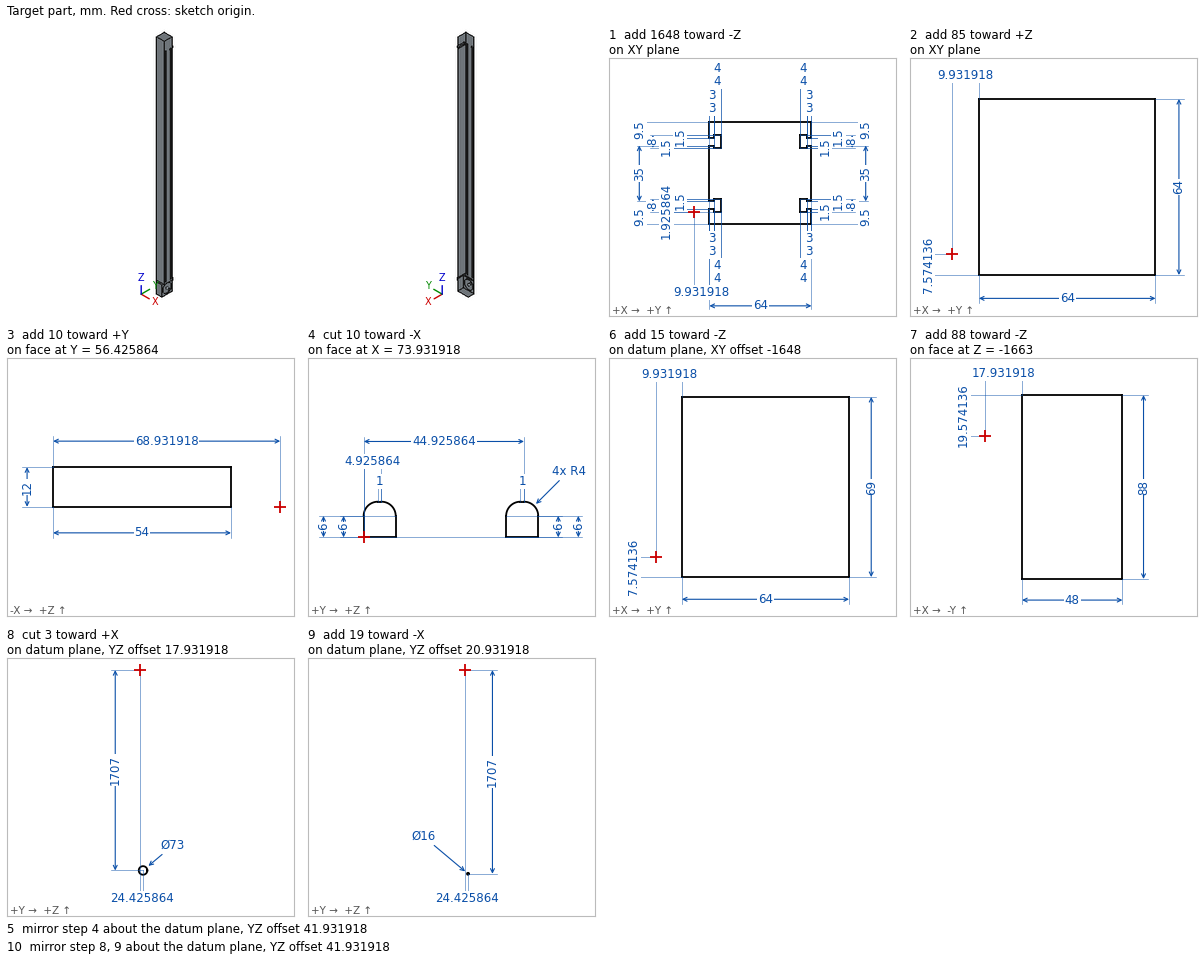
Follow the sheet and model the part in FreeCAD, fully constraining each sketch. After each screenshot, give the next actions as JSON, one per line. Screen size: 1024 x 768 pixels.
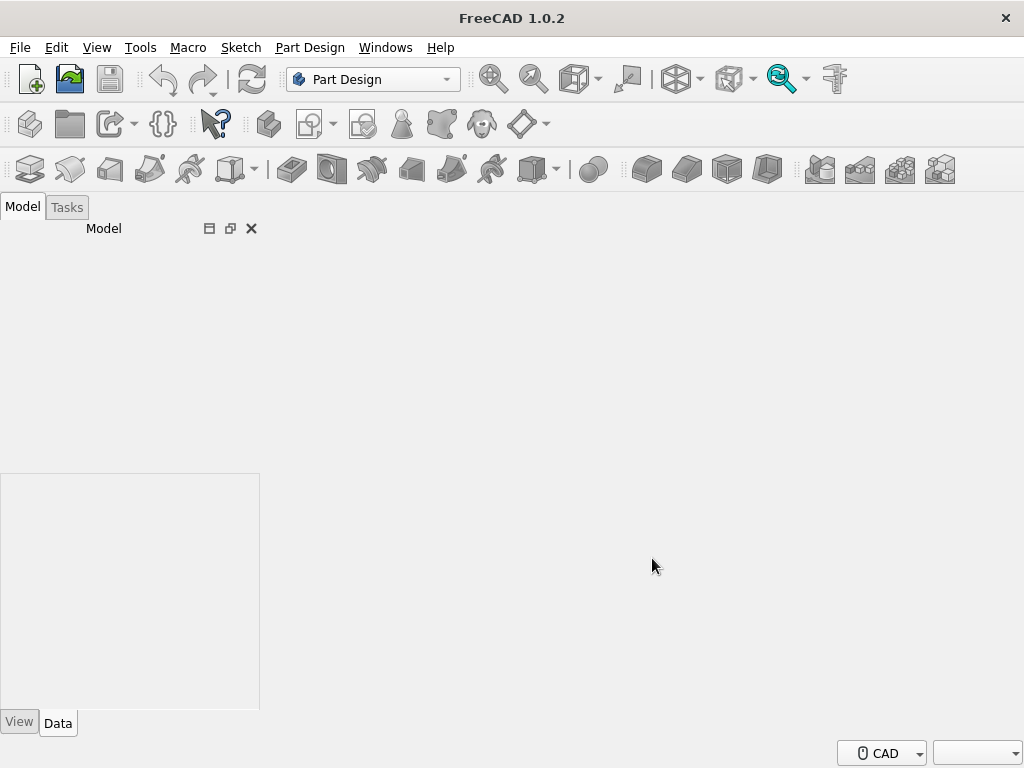
{"action": "left_click", "coordinate": [30, 80]}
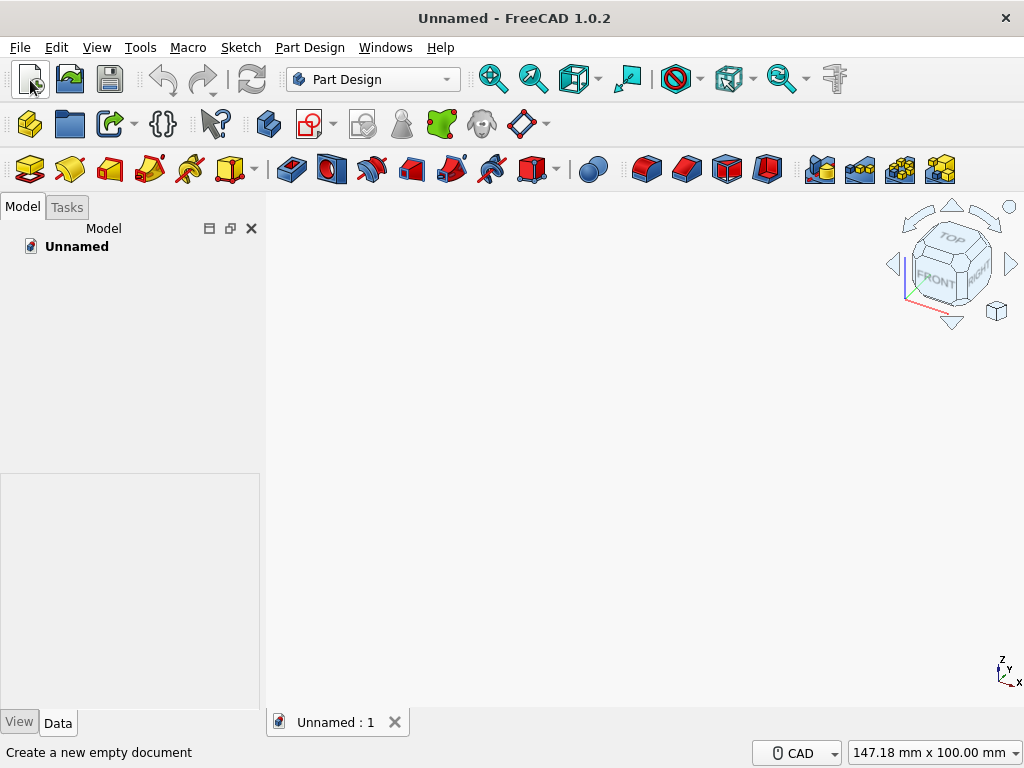
{"action": "left_click", "coordinate": [310, 124]}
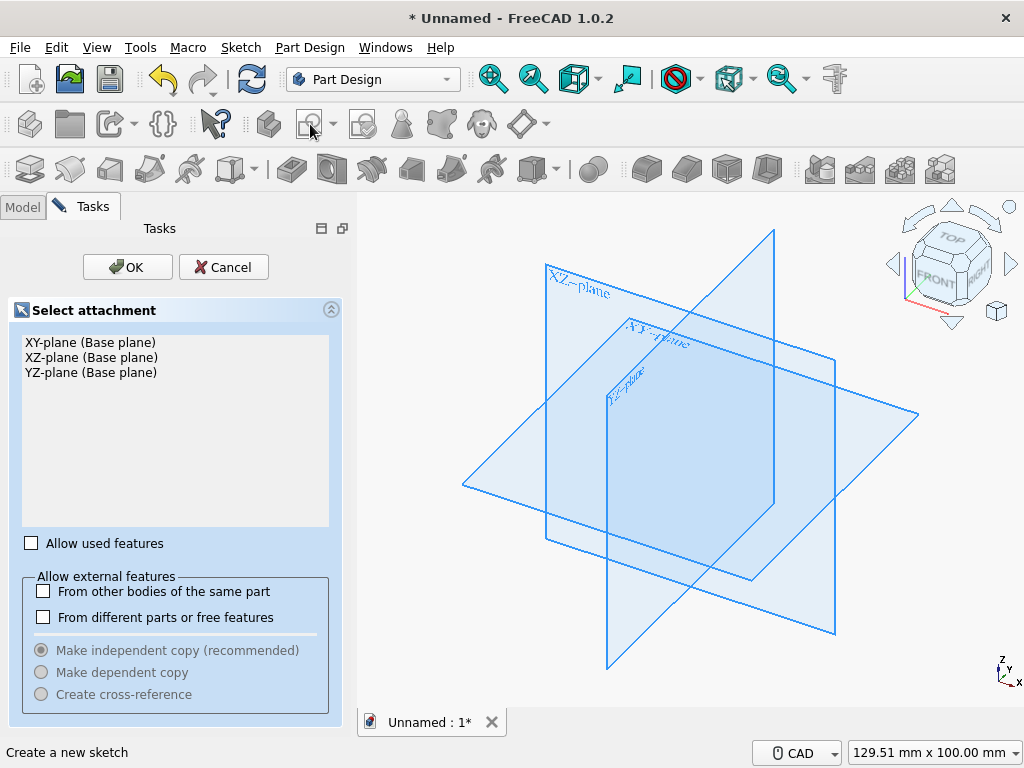
{"action": "left_click", "coordinate": [82, 342]}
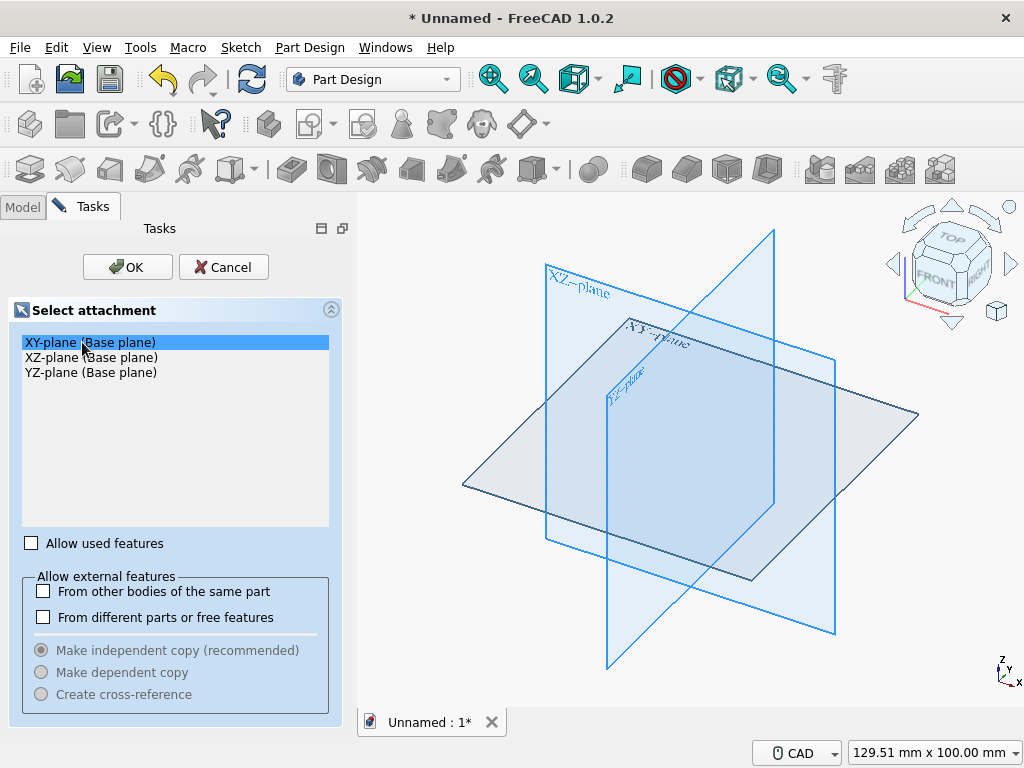
{"action": "left_click", "coordinate": [128, 267]}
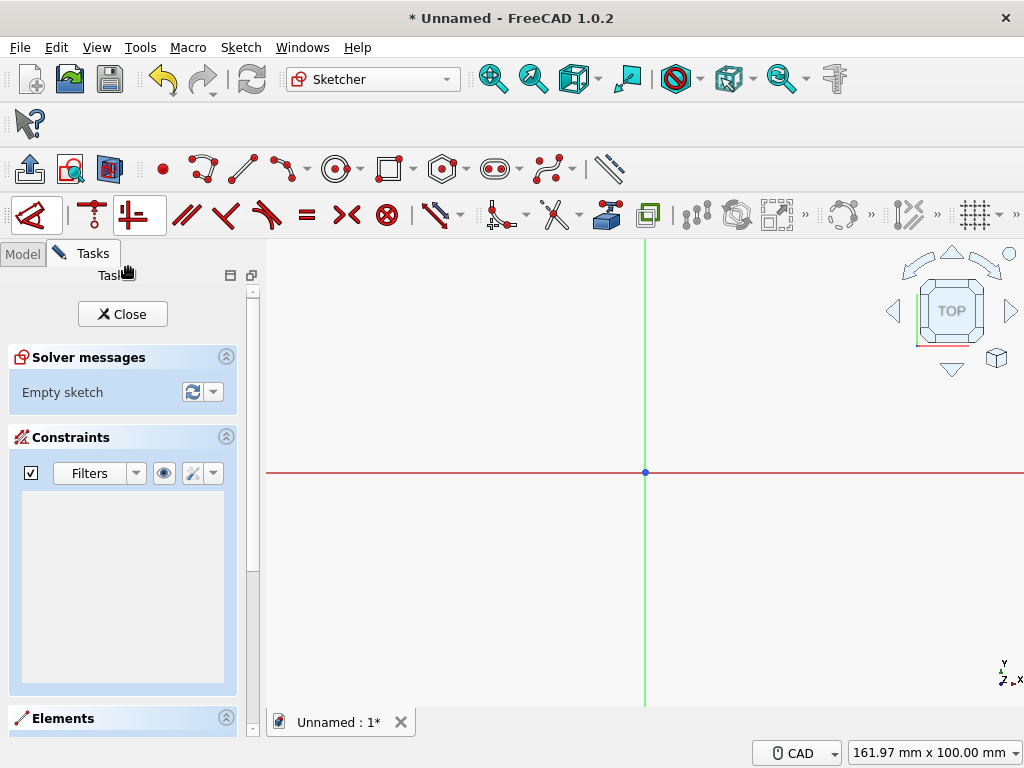
{"action": "scroll", "coordinate": [294, 679], "scroll_direction": "down", "scroll_amount": 2}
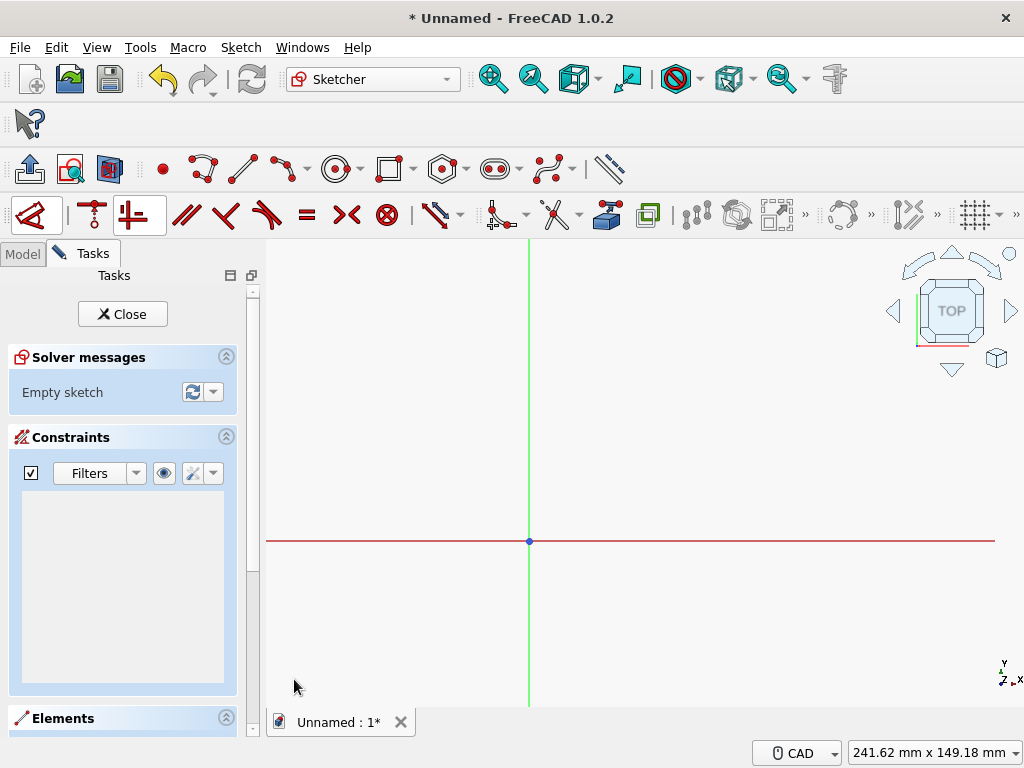
{"action": "scroll", "coordinate": [785, 448], "scroll_direction": "up", "scroll_amount": 2}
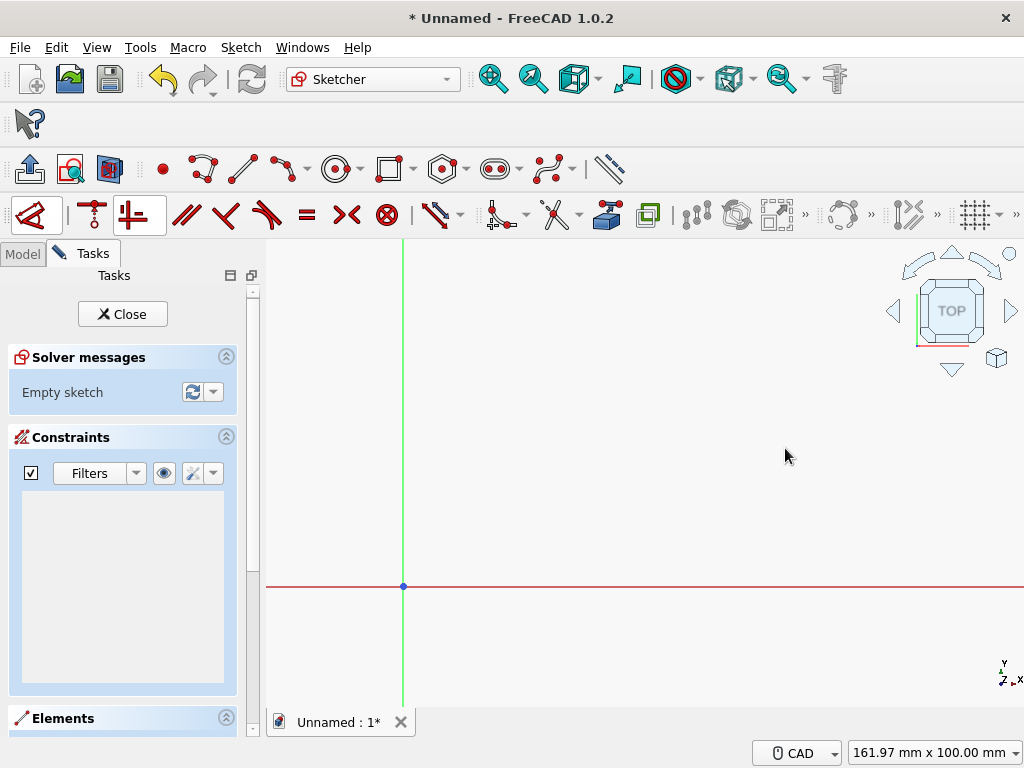
{"action": "left_click", "coordinate": [204, 170]}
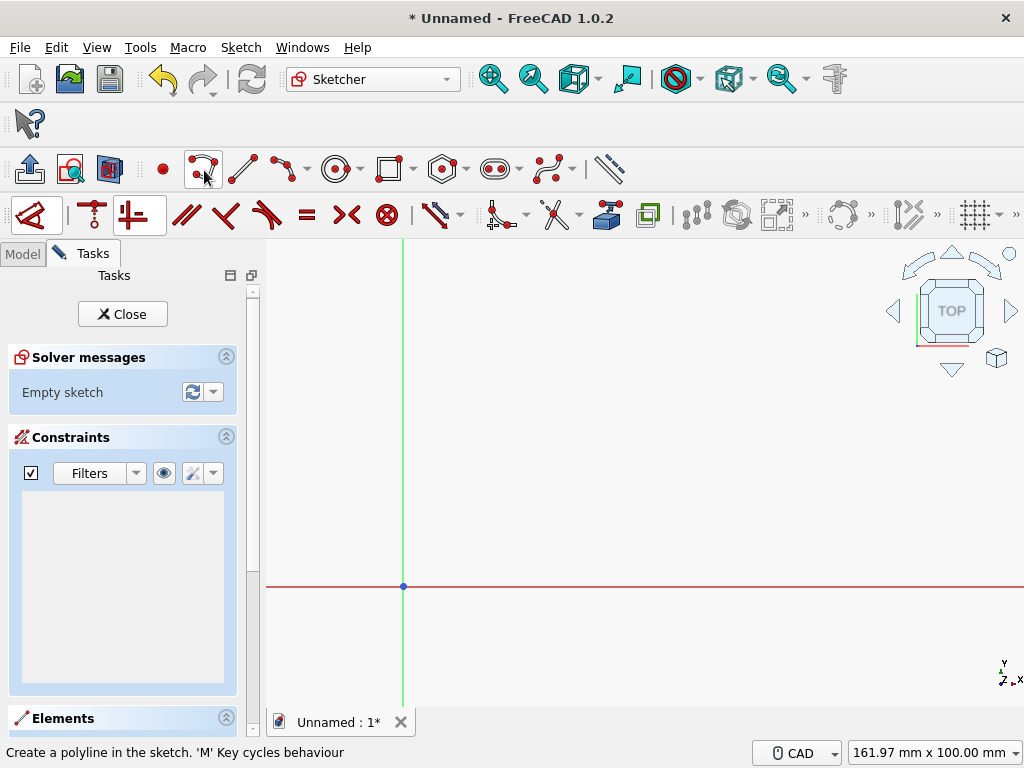
{"action": "scroll", "coordinate": [450, 578], "scroll_direction": "up", "scroll_amount": 3}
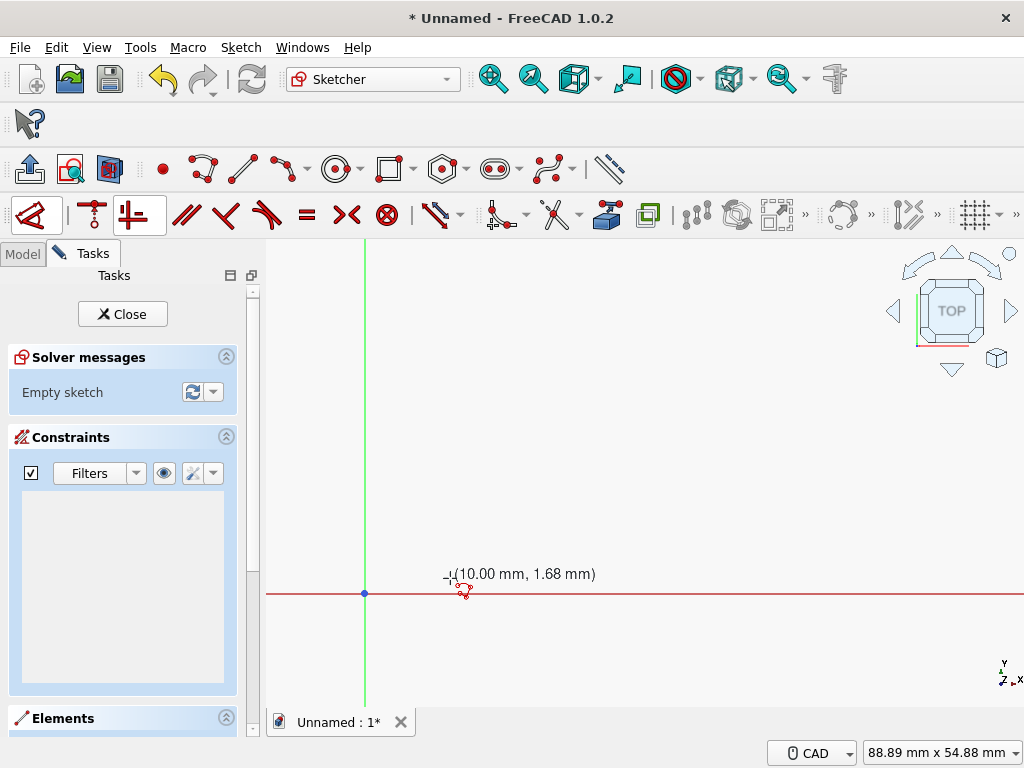
{"action": "left_click", "coordinate": [449, 577]}
{"action": "left_click", "coordinate": [449, 658]}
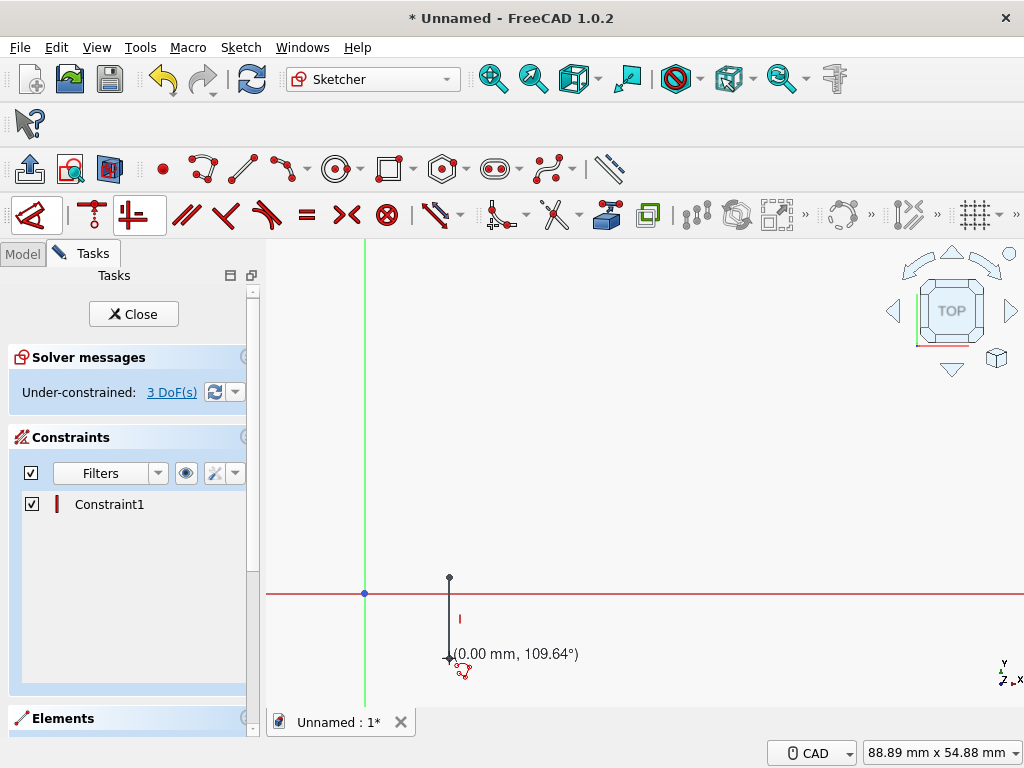
{"action": "scroll", "coordinate": [451, 580], "scroll_direction": "down", "scroll_amount": 3}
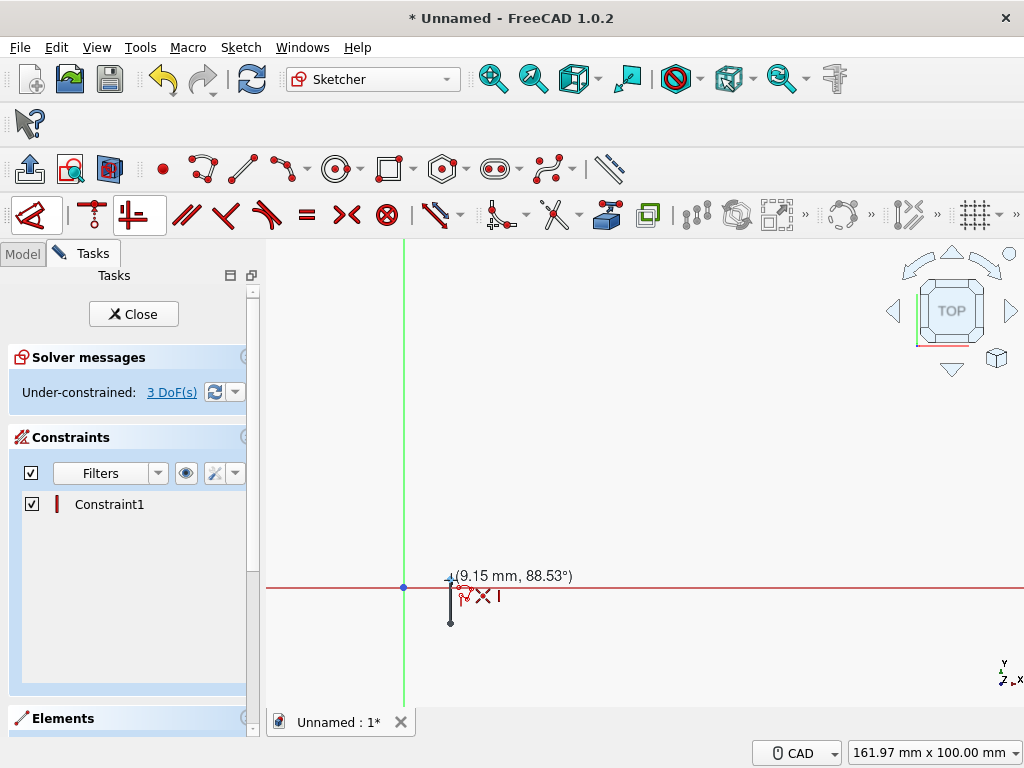
{"action": "left_click", "coordinate": [750, 623]}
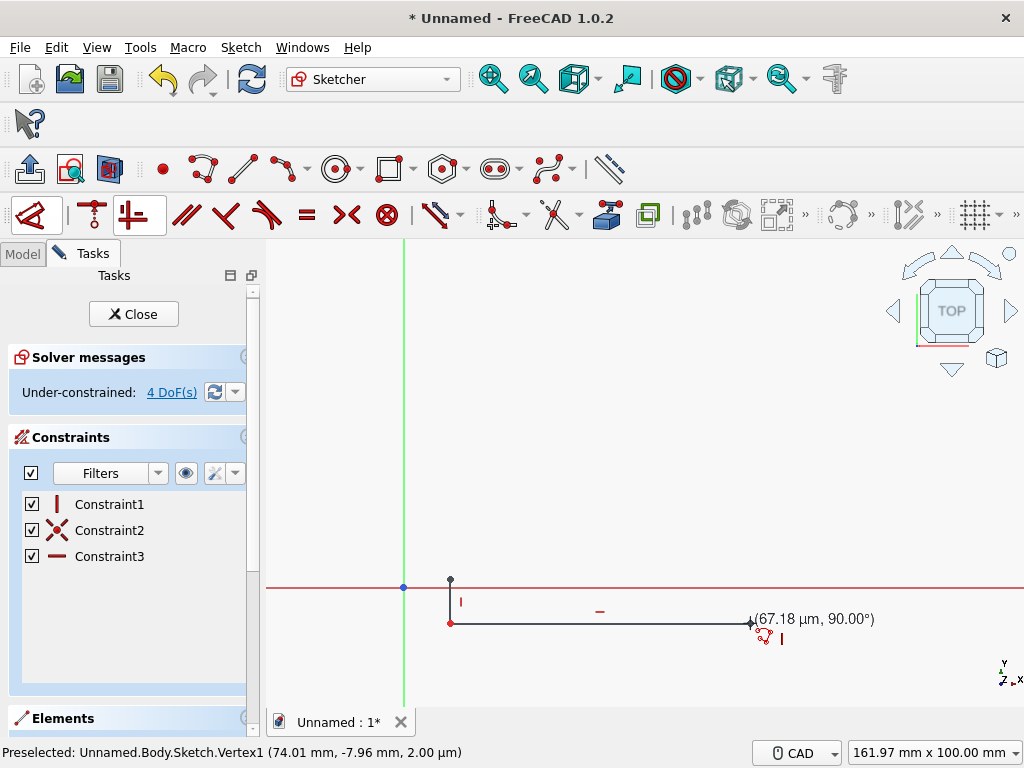
{"action": "scroll", "coordinate": [750, 579], "scroll_direction": "up", "scroll_amount": 3}